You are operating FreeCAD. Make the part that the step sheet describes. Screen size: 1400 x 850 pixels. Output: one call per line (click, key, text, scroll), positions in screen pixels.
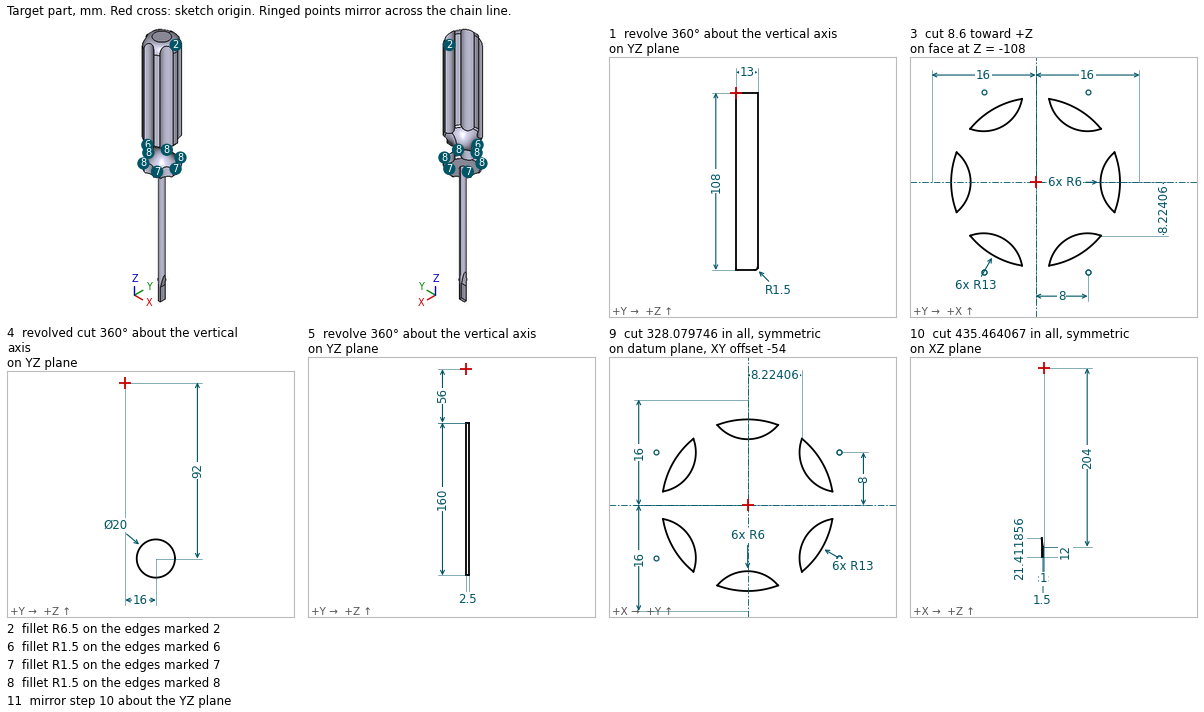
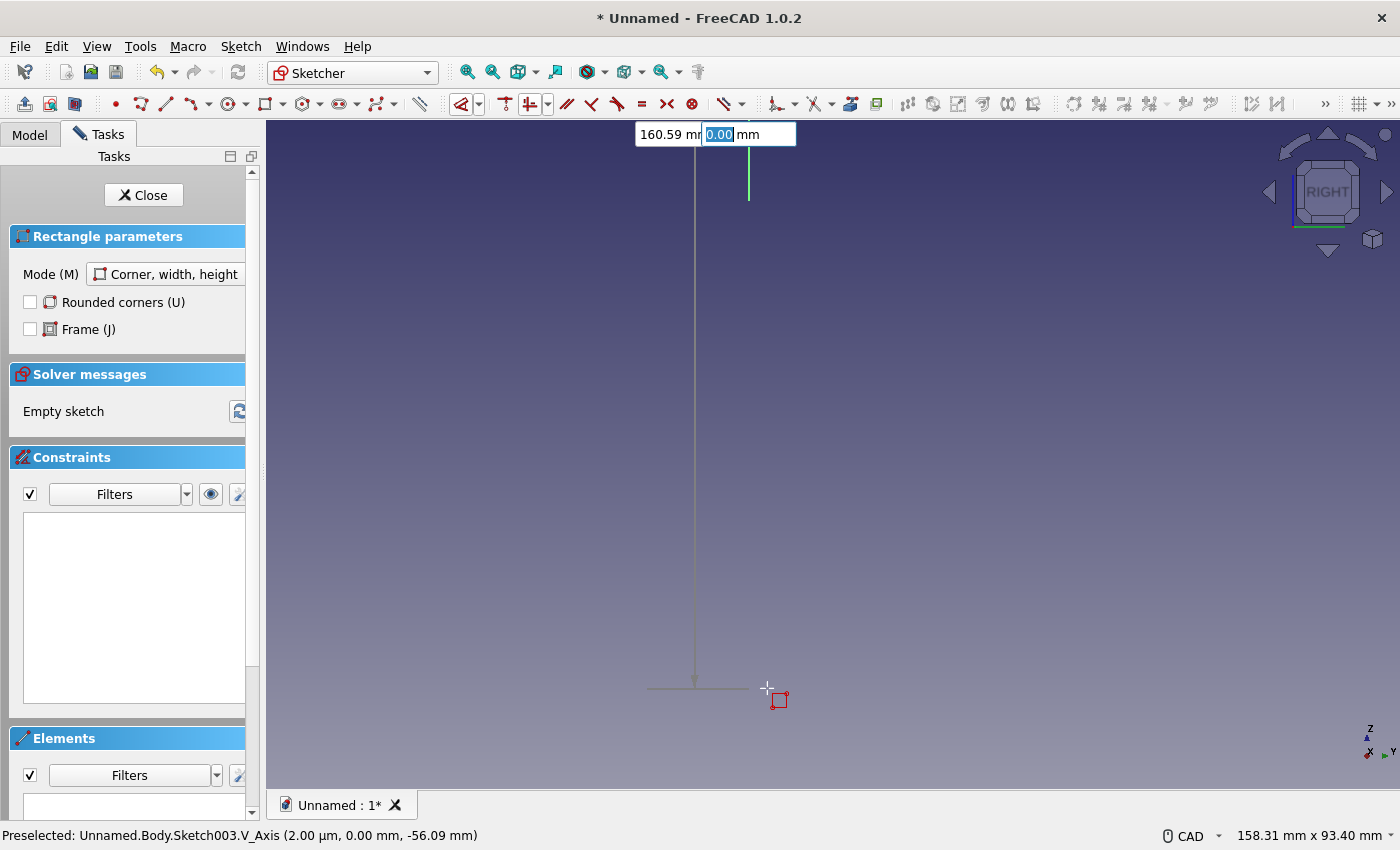
click(767, 684)
key(Escape)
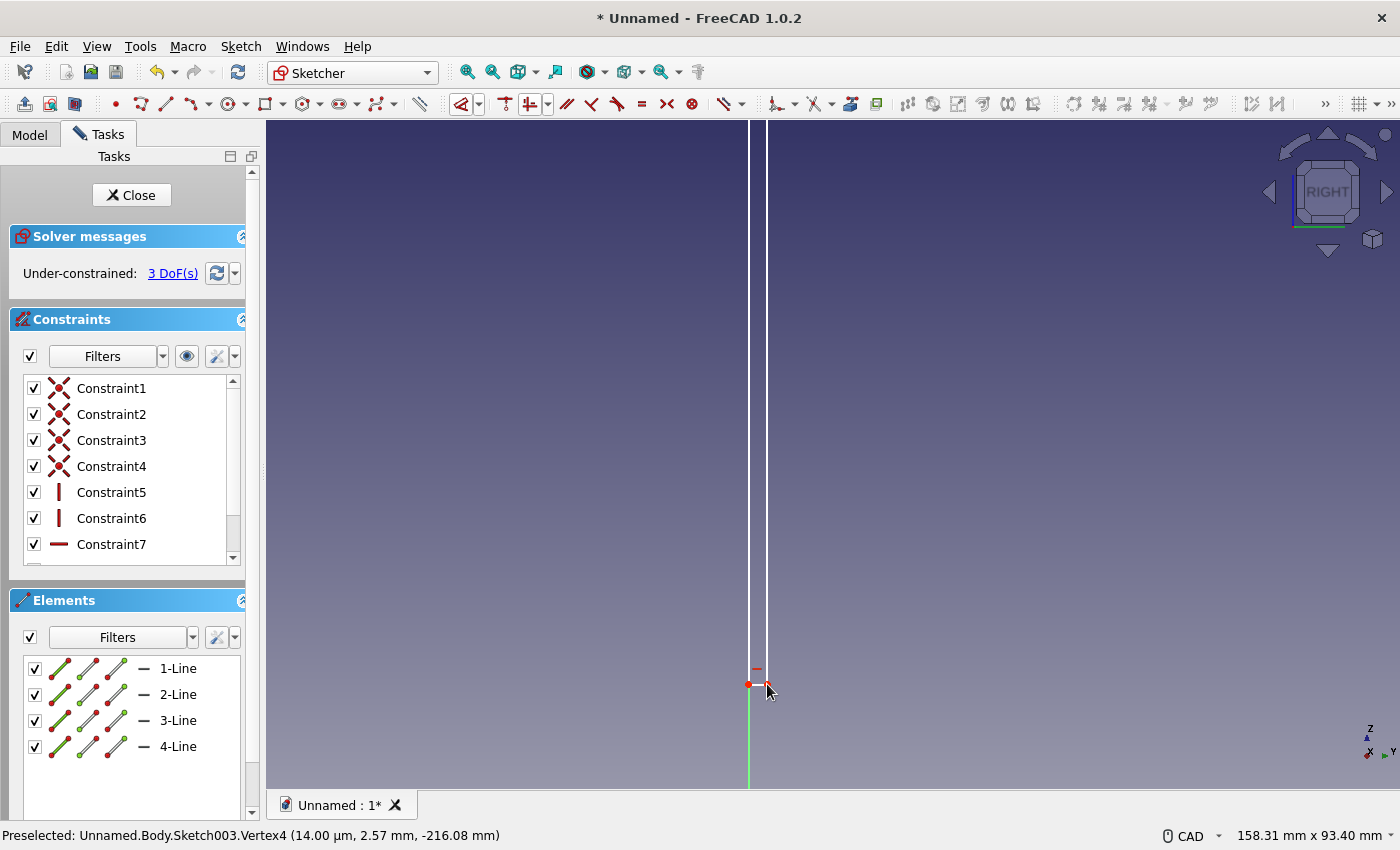
key(d)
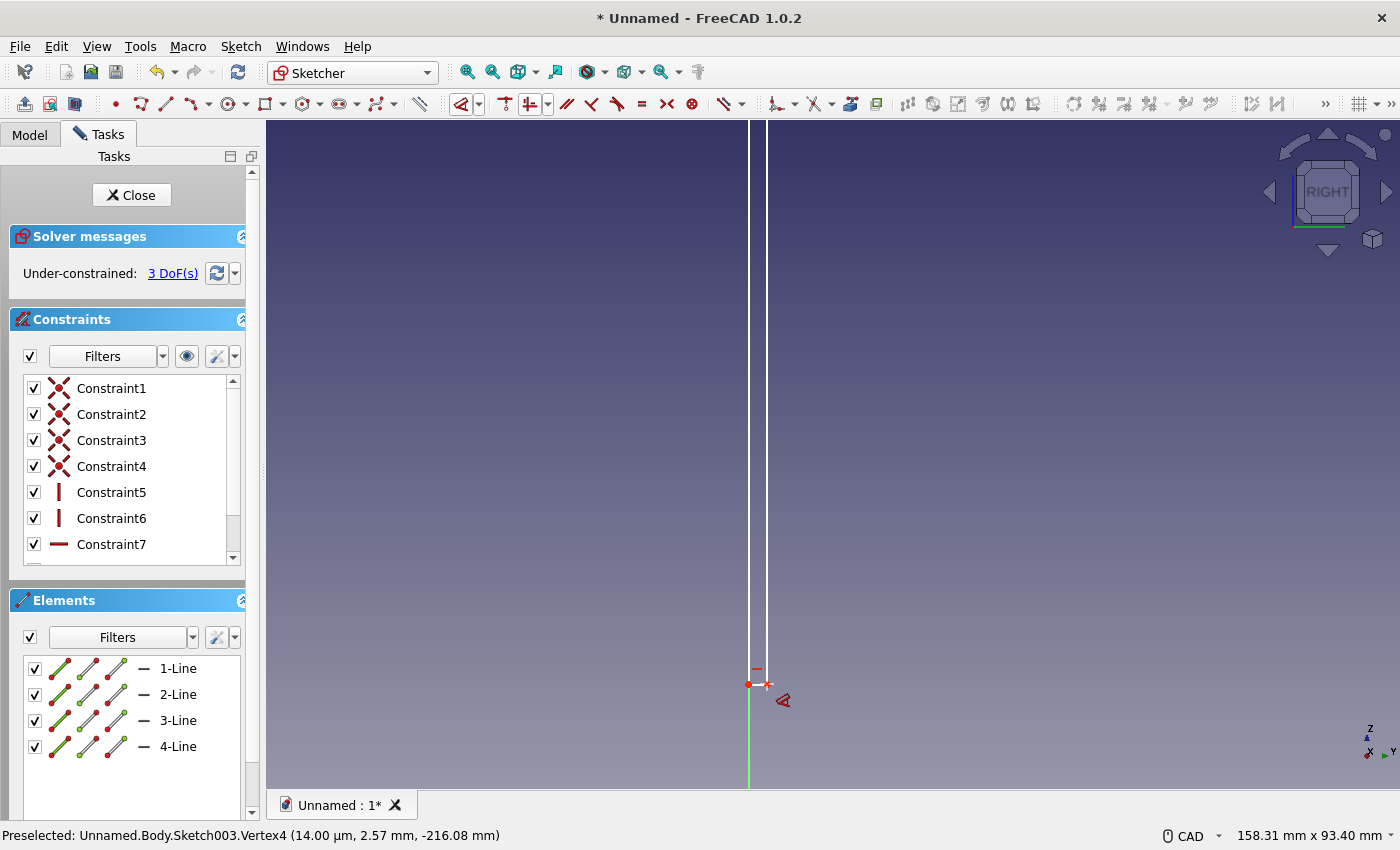
click(749, 341)
click(715, 417)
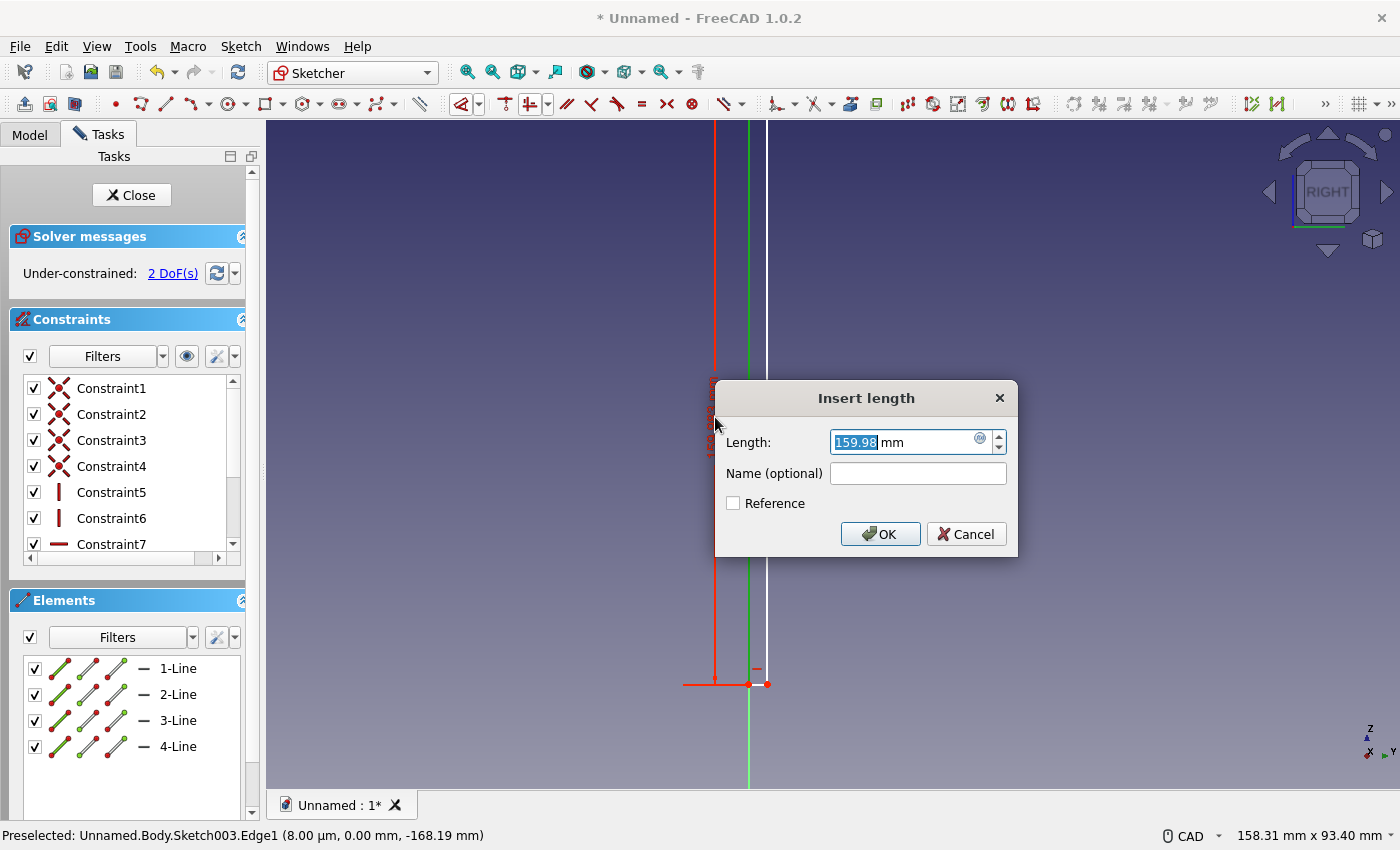
text(160)
key(Return)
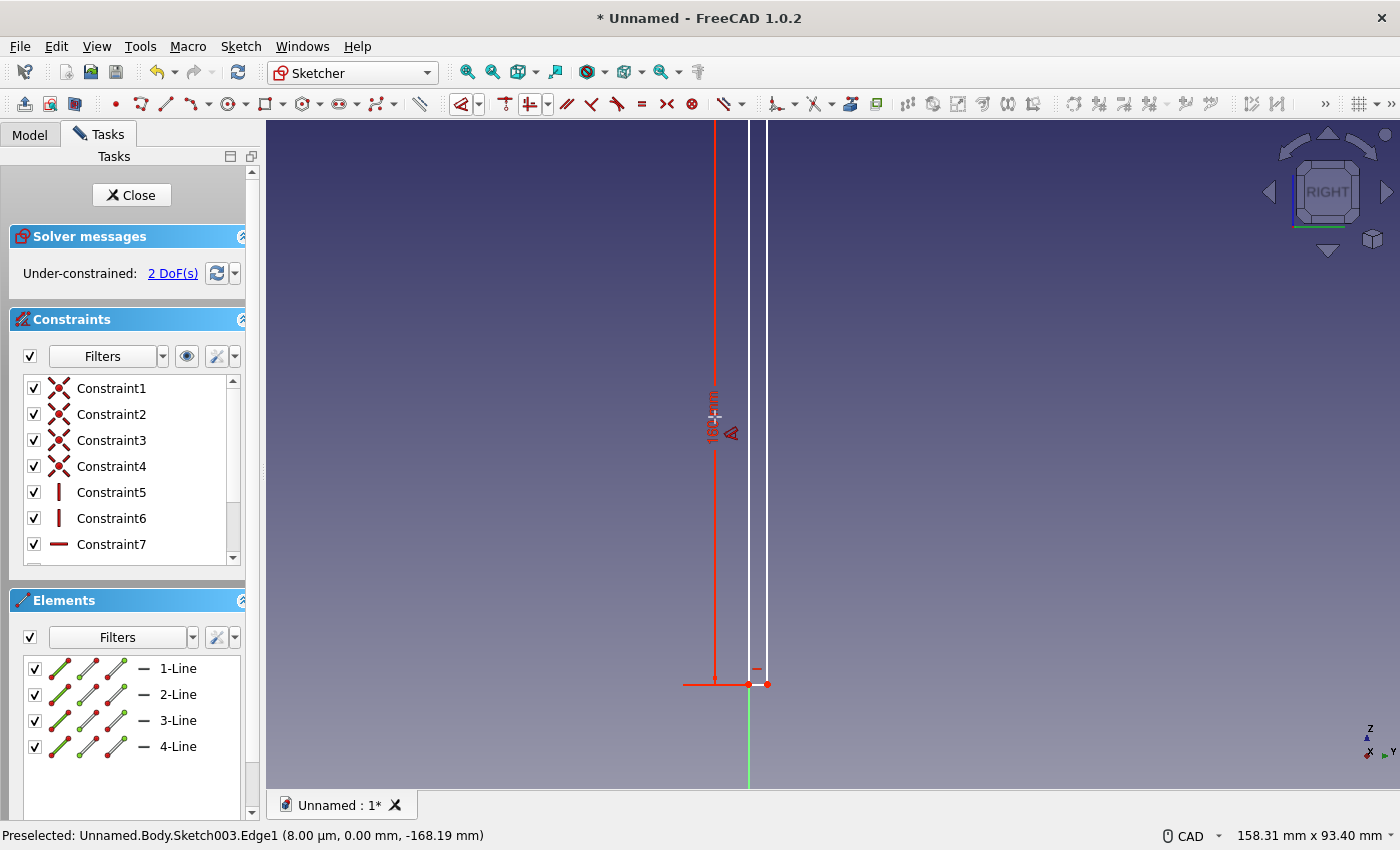
scroll(758, 685, up, 4)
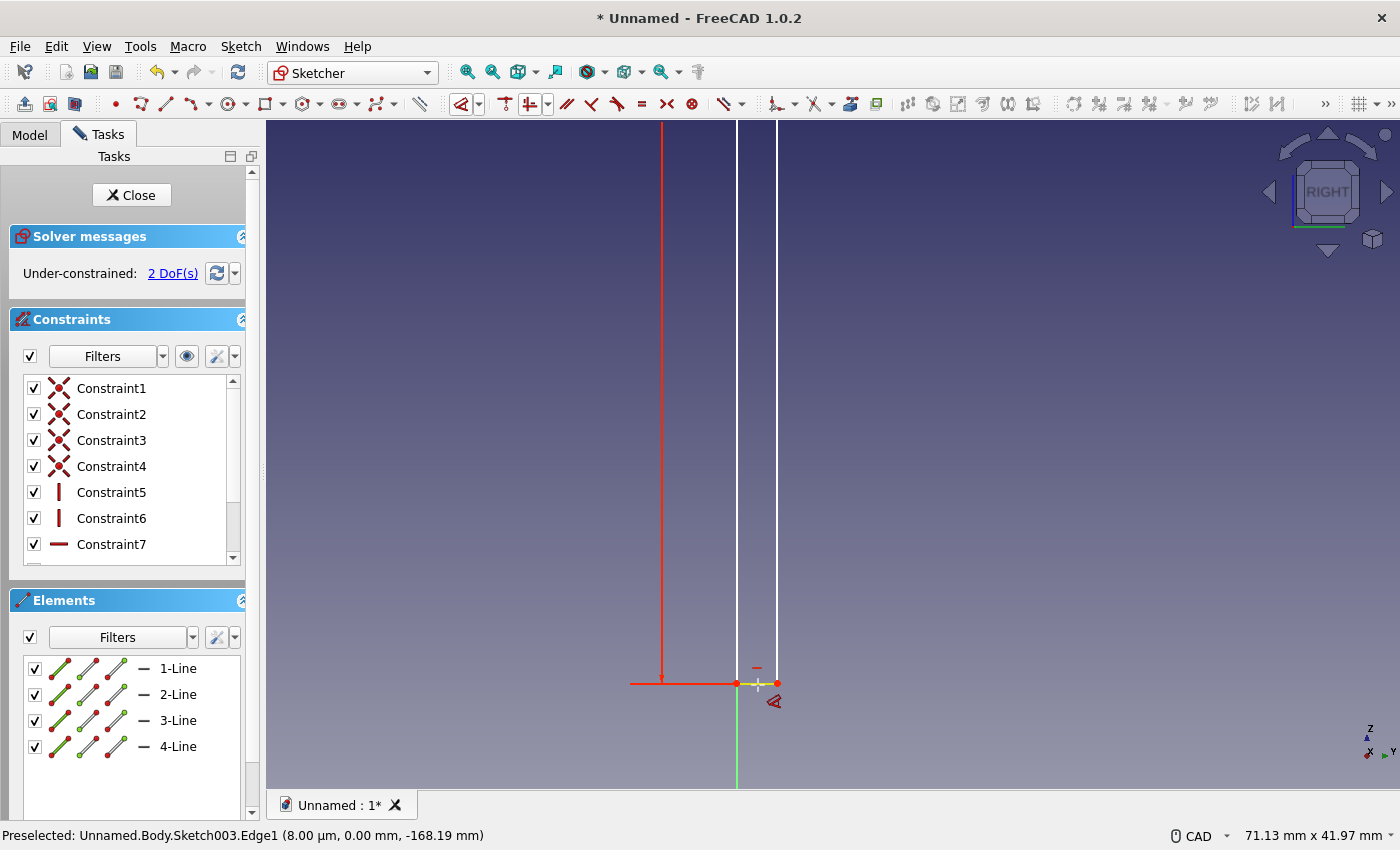
click(757, 684)
click(757, 718)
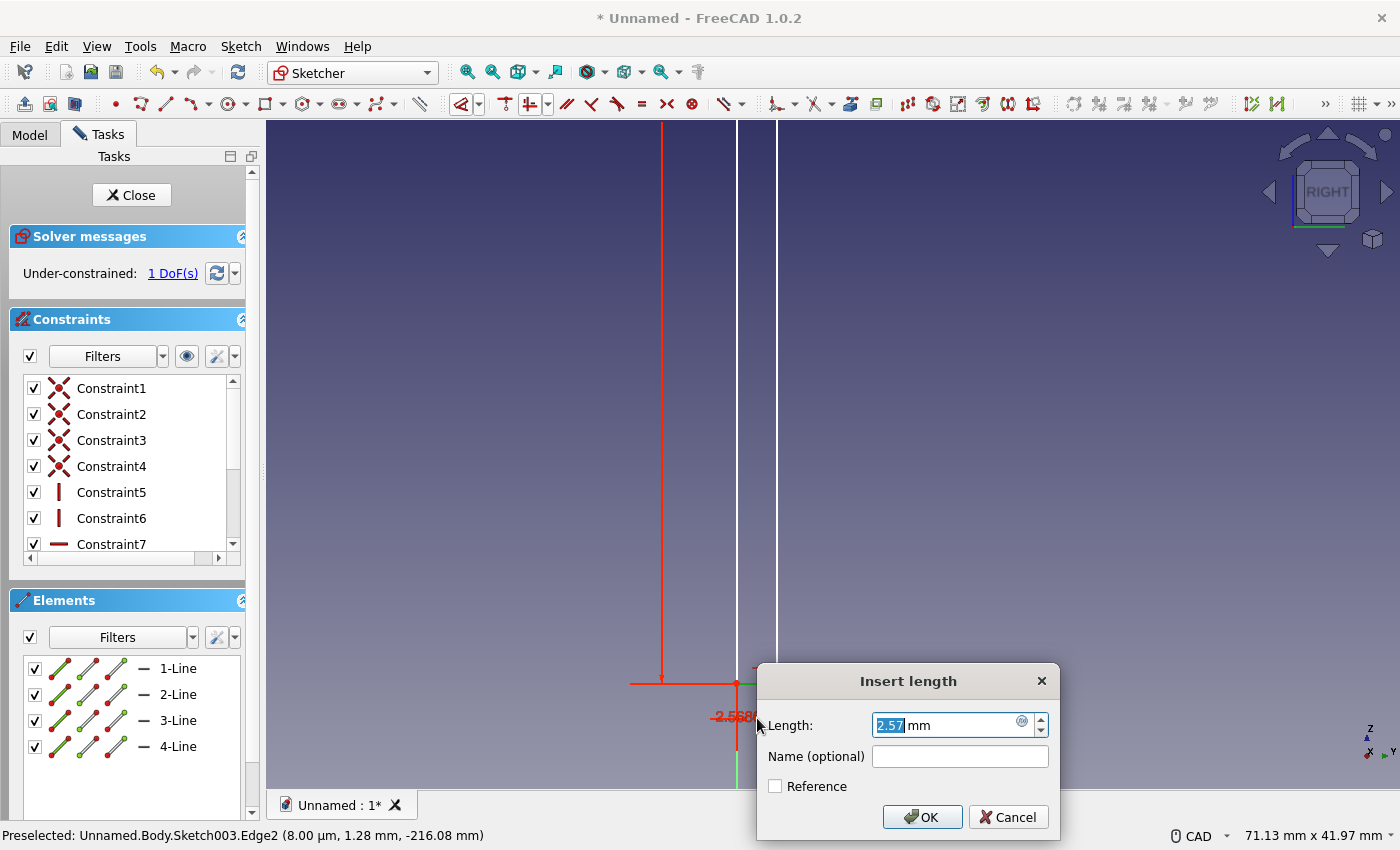
text(2.5)
key(Return)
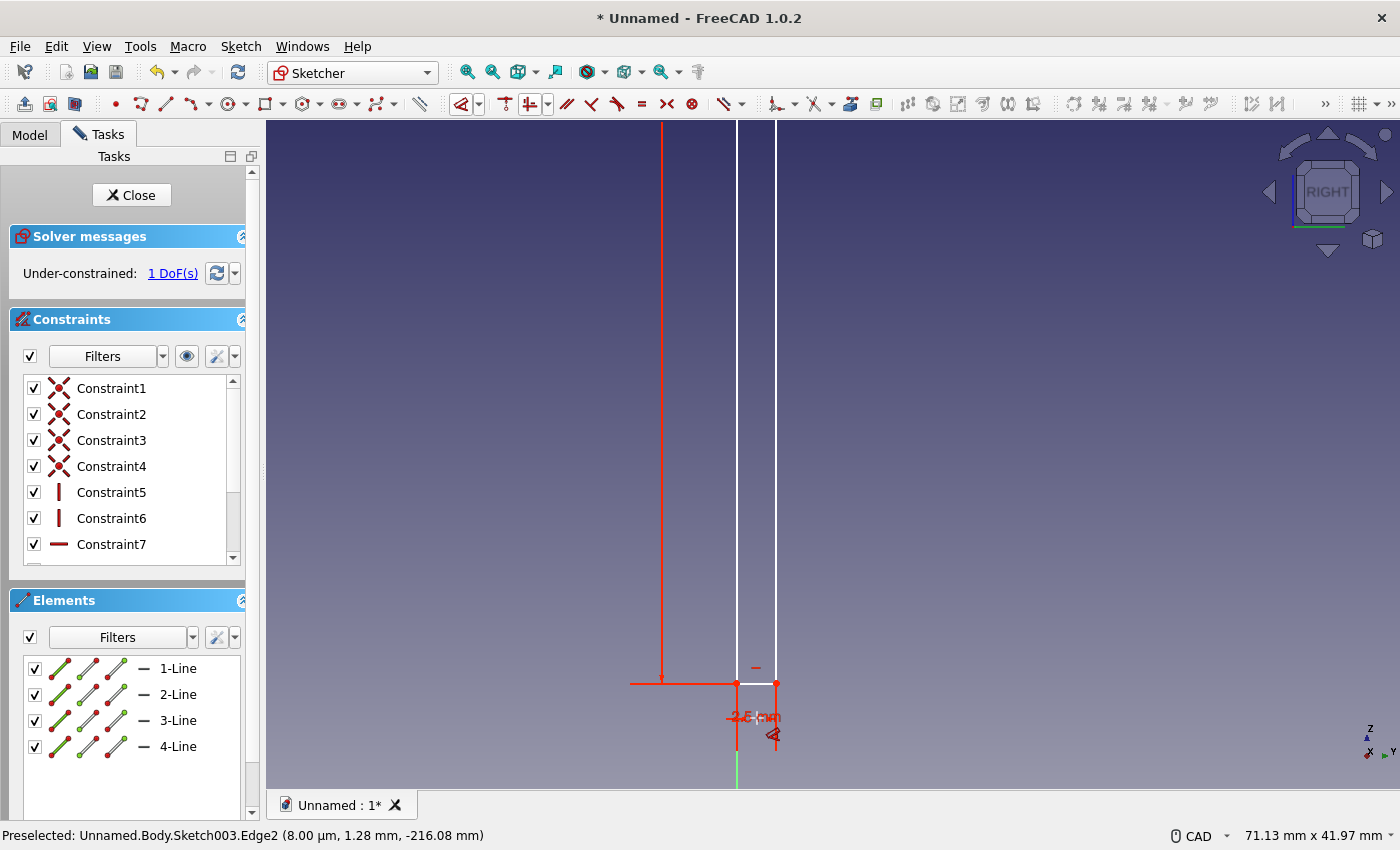
scroll(766, 688, down, 10)